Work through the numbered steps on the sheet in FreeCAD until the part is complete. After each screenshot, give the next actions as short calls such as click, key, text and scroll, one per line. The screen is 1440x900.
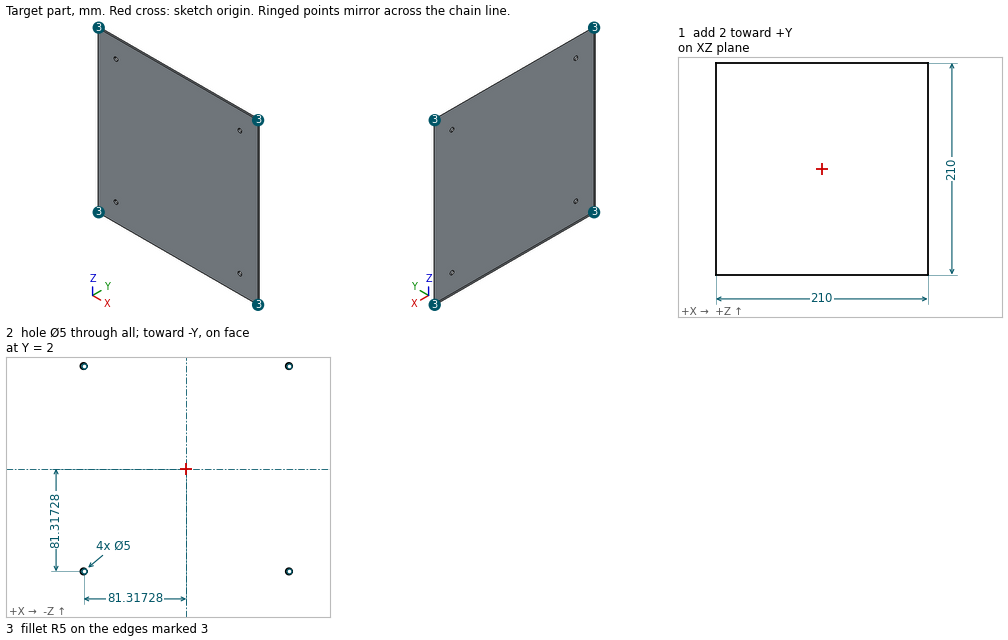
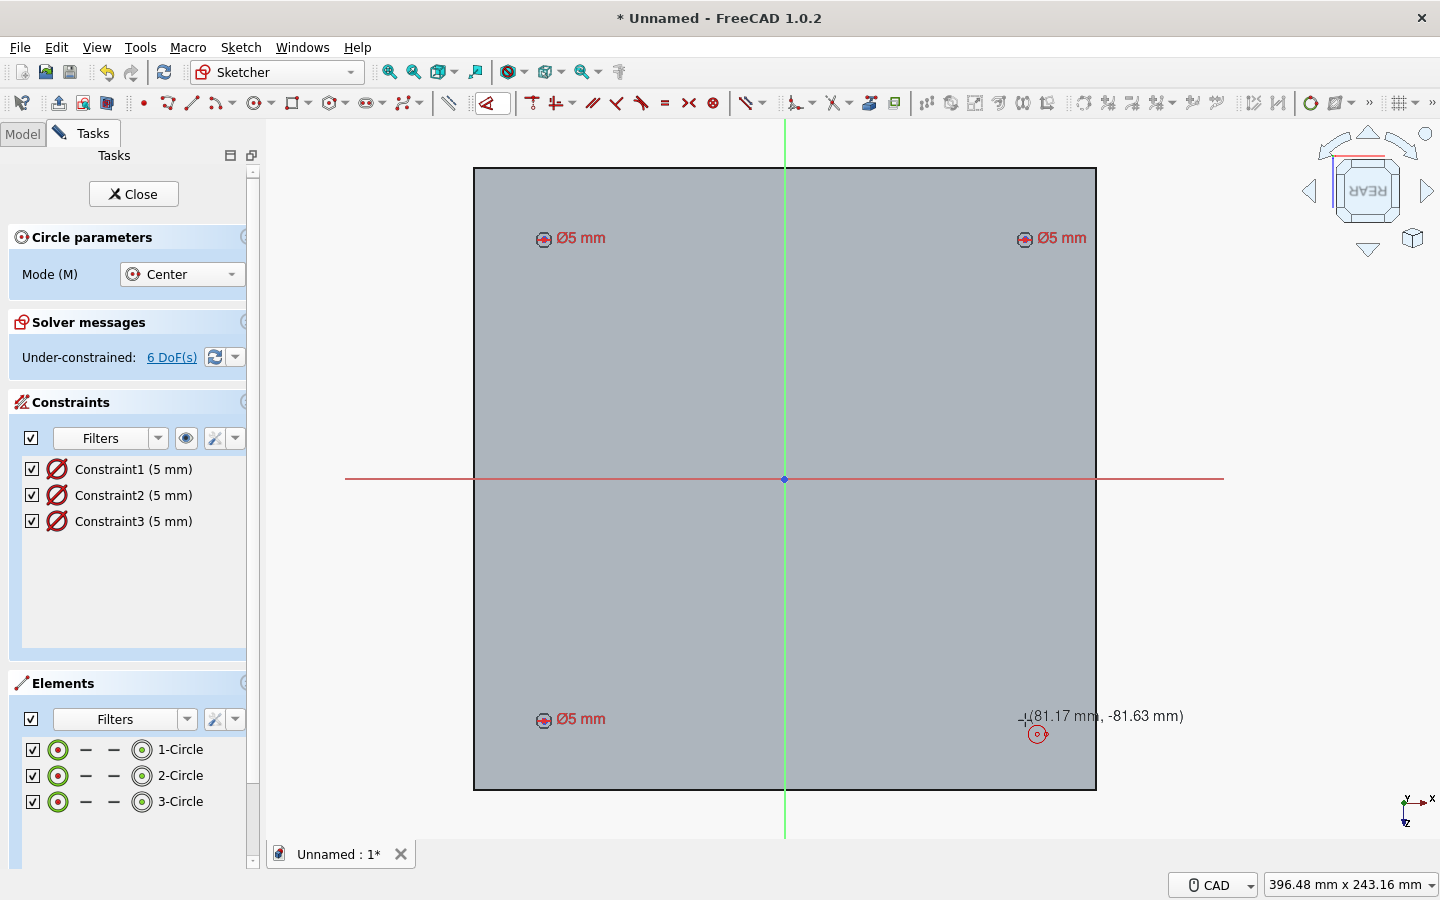
click(1025, 720)
move(1031, 715)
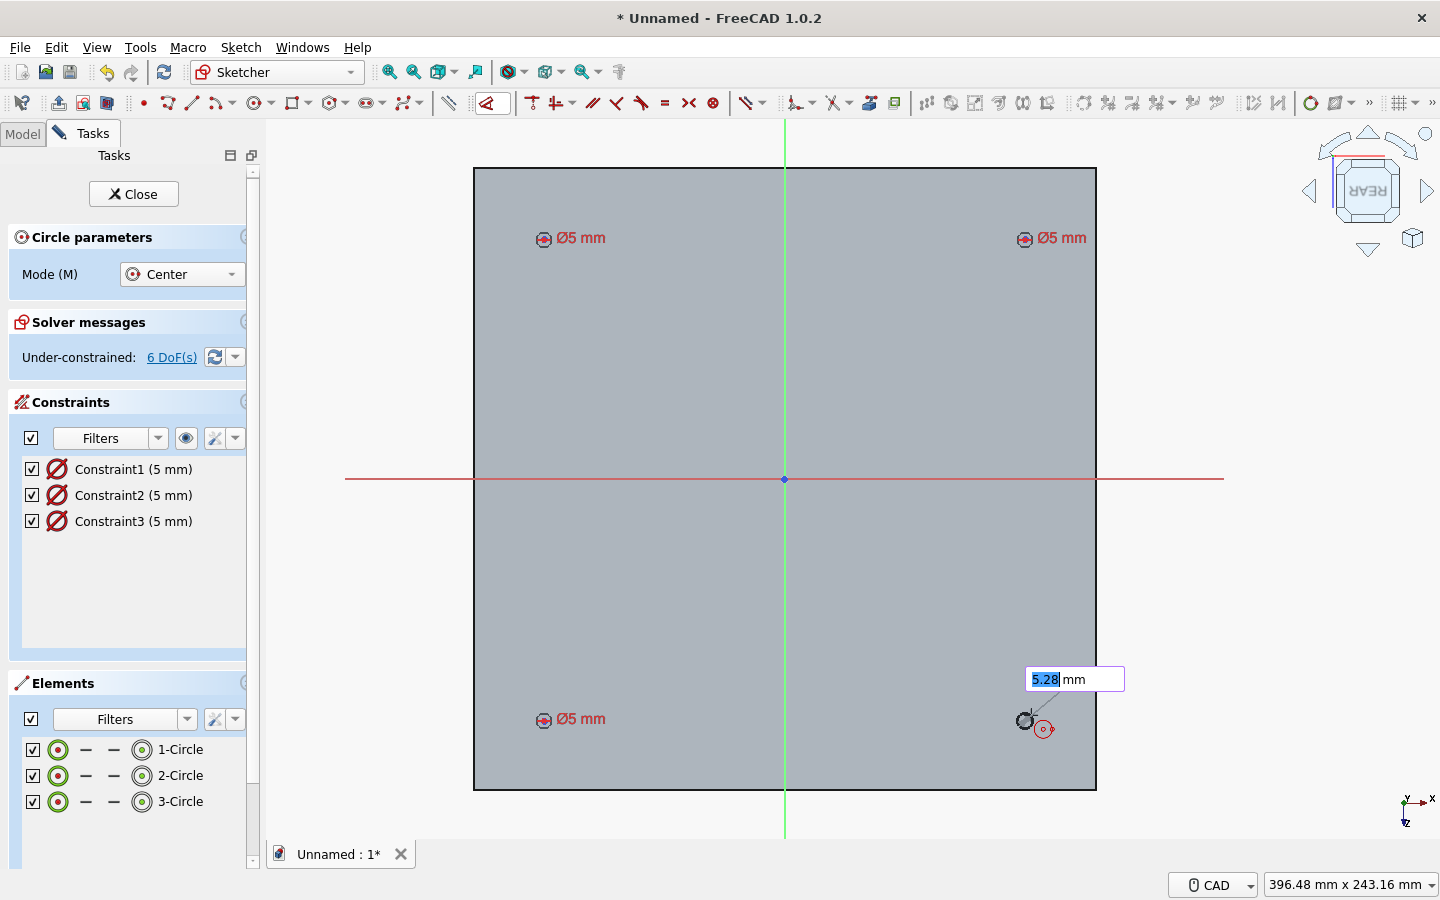
text(5)
key(Return)
key(Escape)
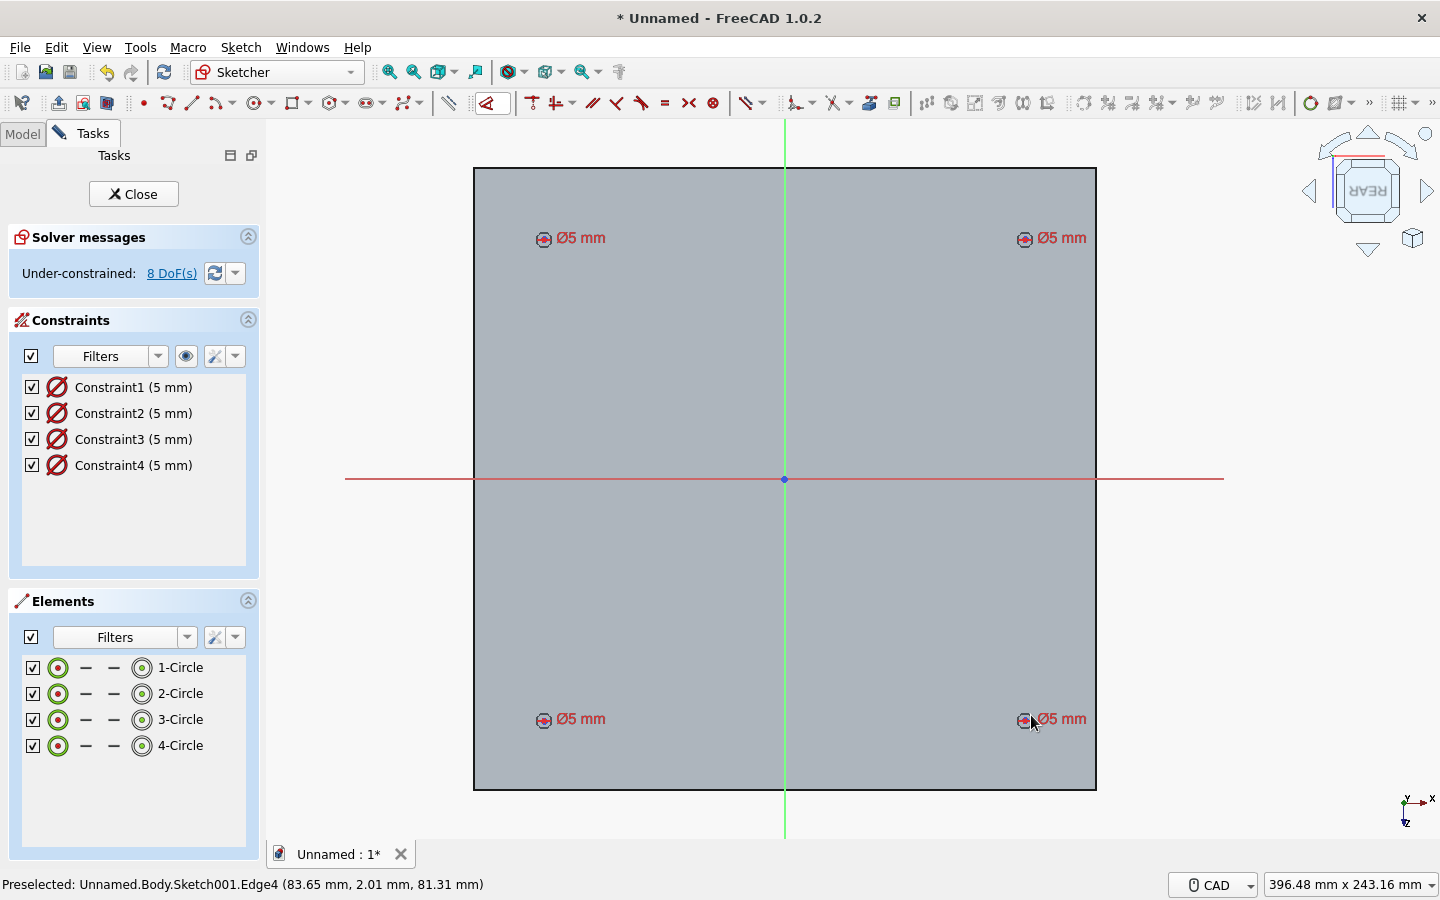
click(544, 721)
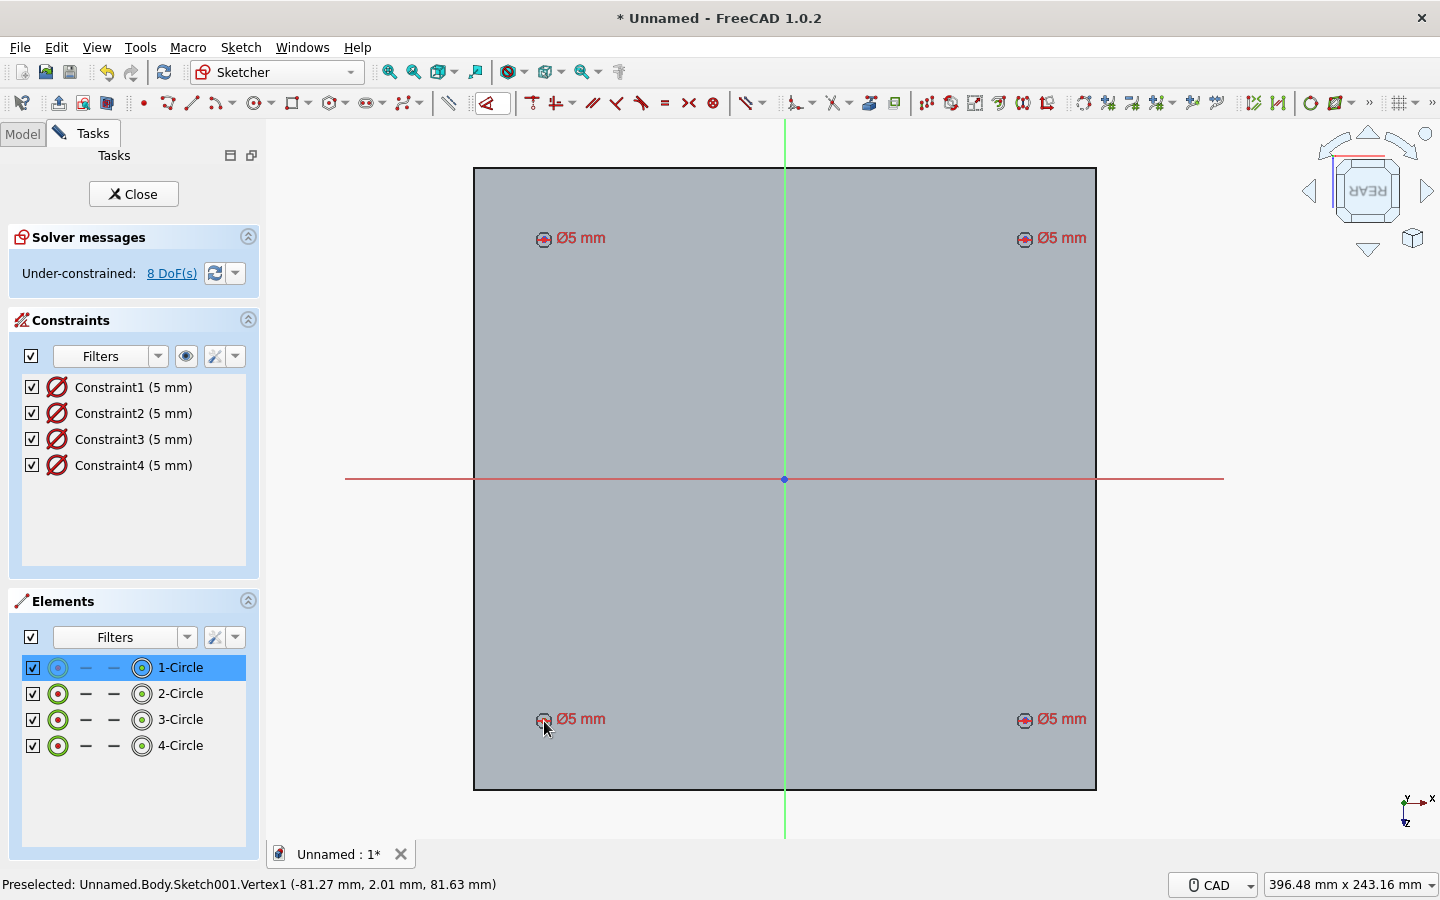
click(544, 240)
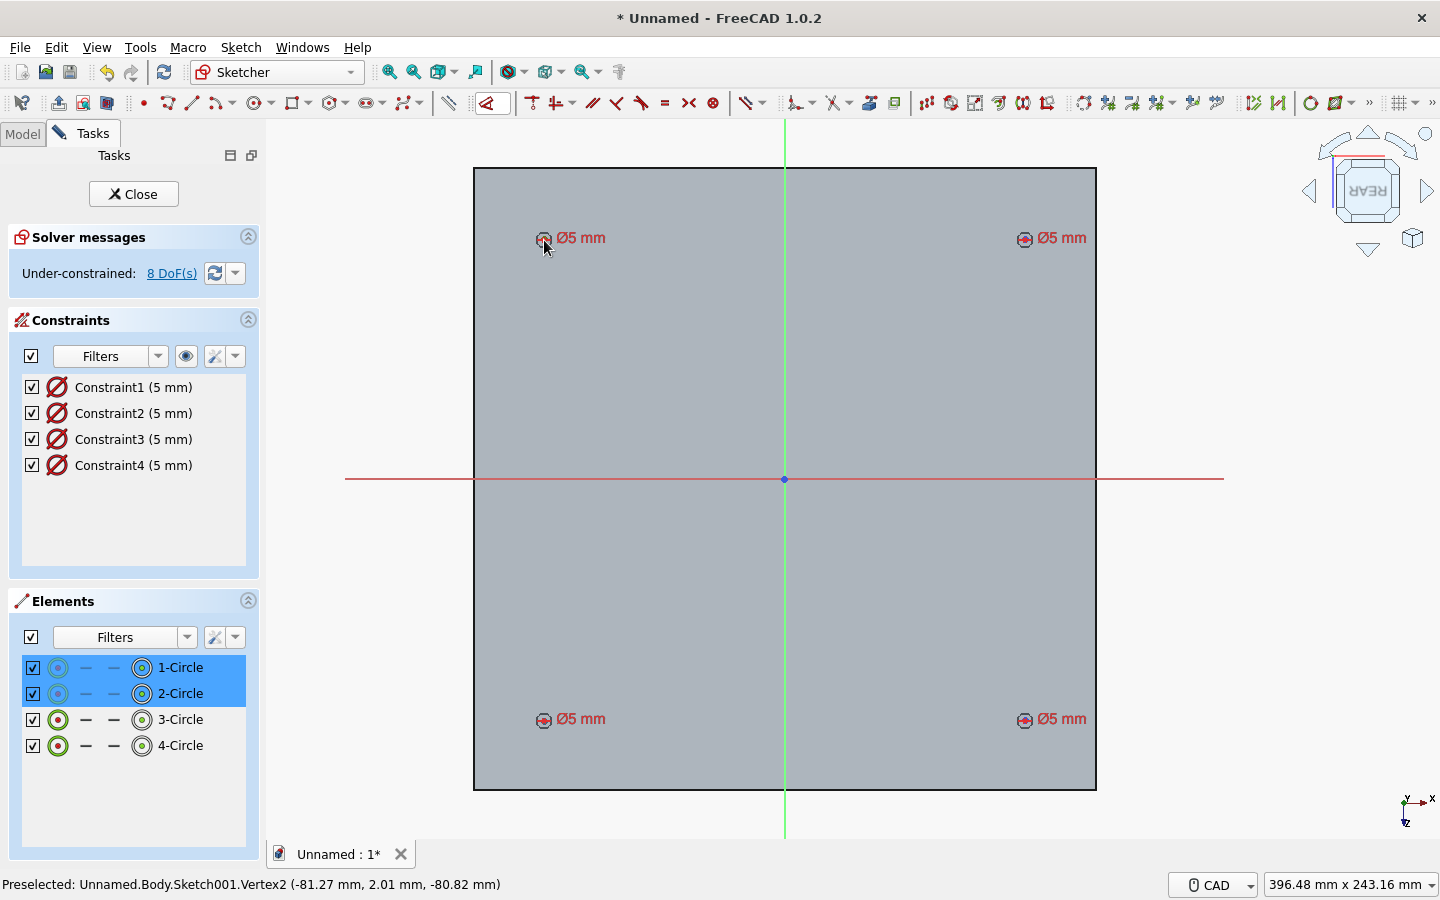
click(364, 479)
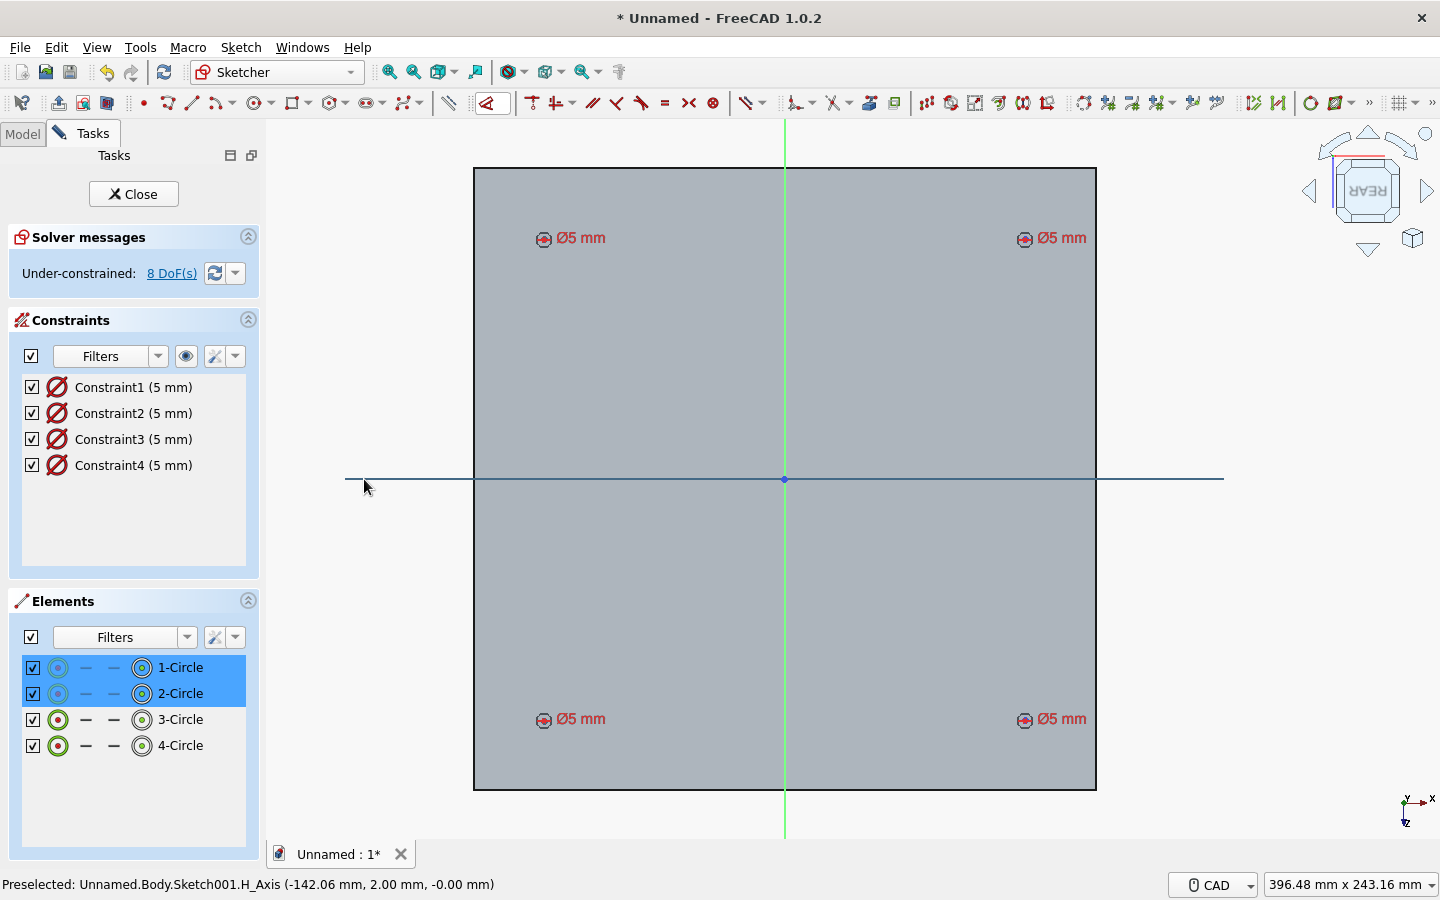
click(690, 104)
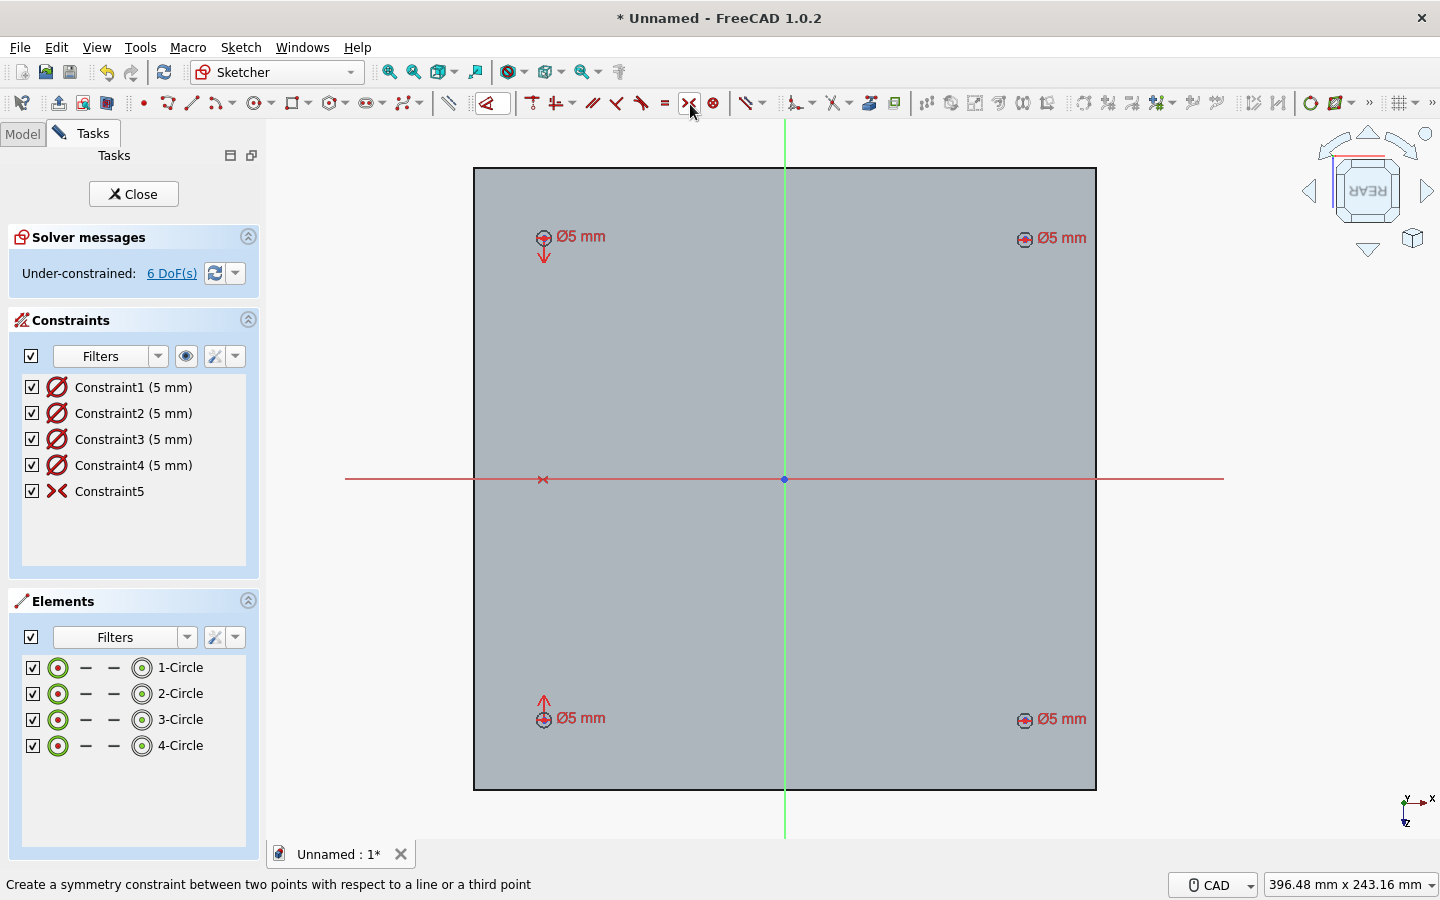
click(544, 238)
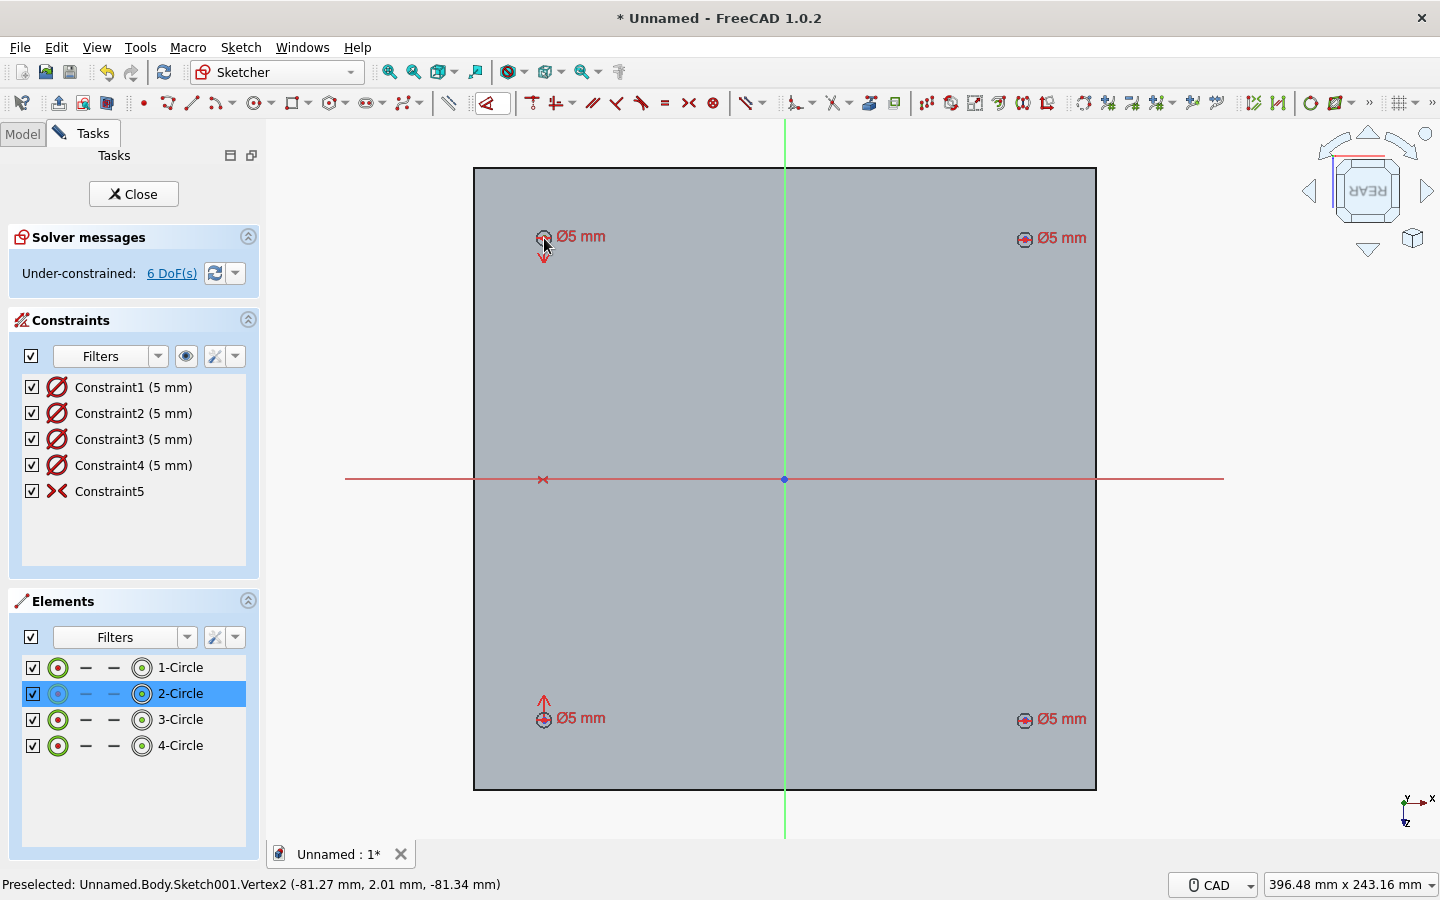
click(1025, 240)